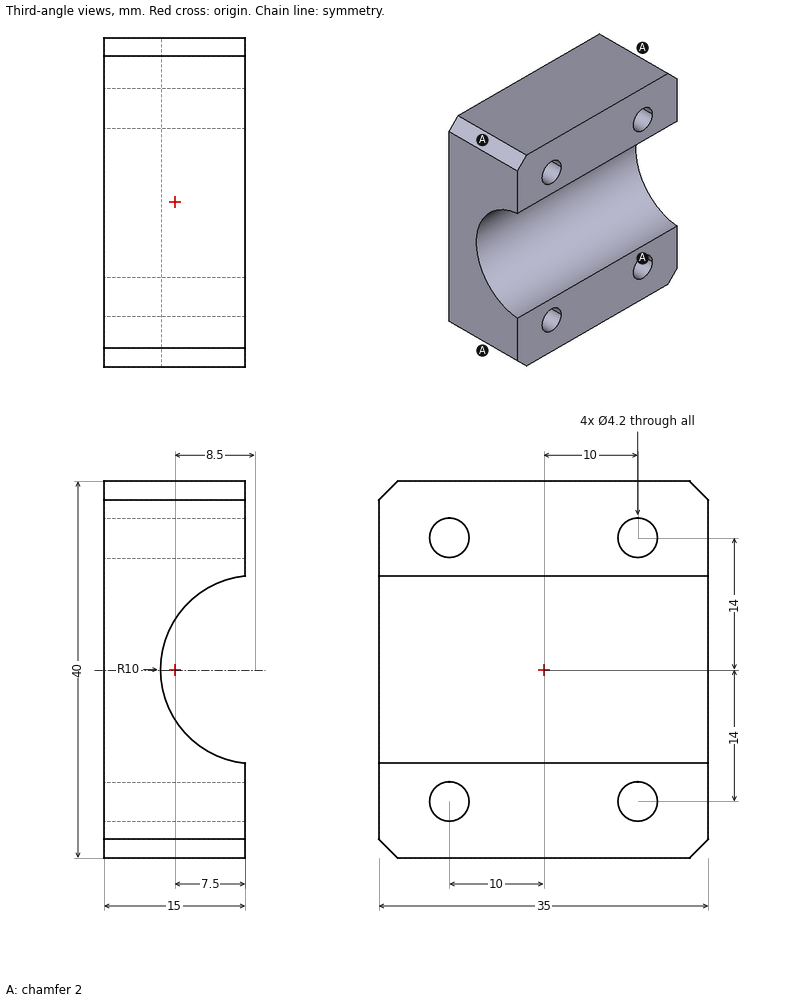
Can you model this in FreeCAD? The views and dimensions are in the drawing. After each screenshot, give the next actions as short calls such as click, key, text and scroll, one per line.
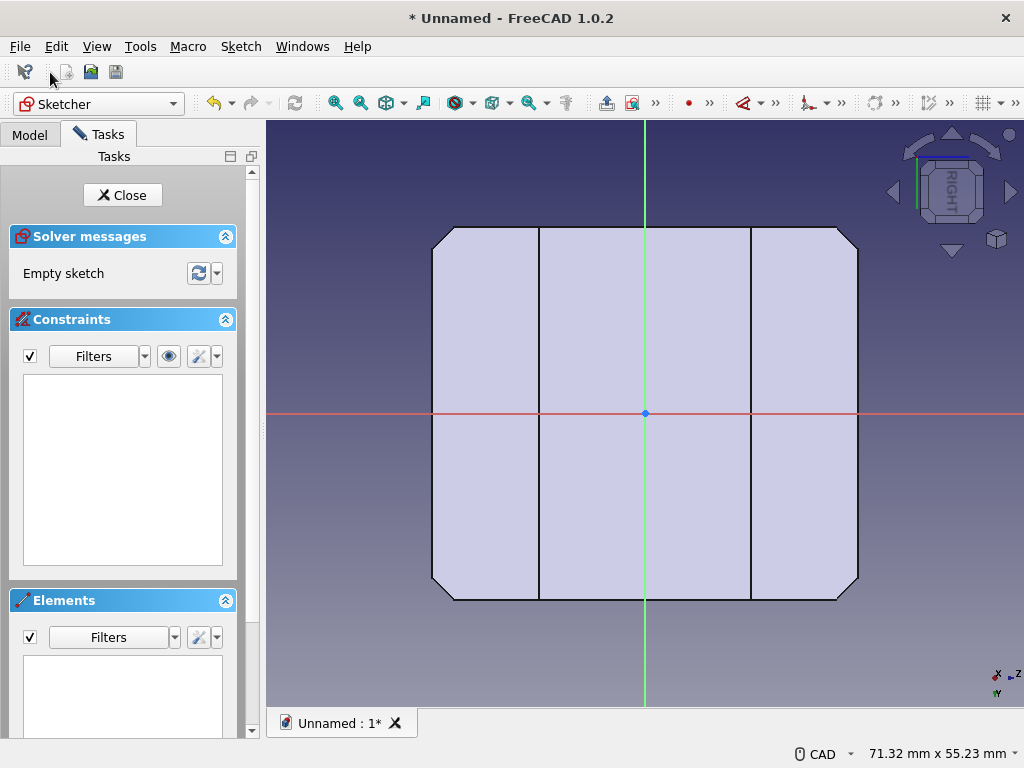
key(g)
key(c)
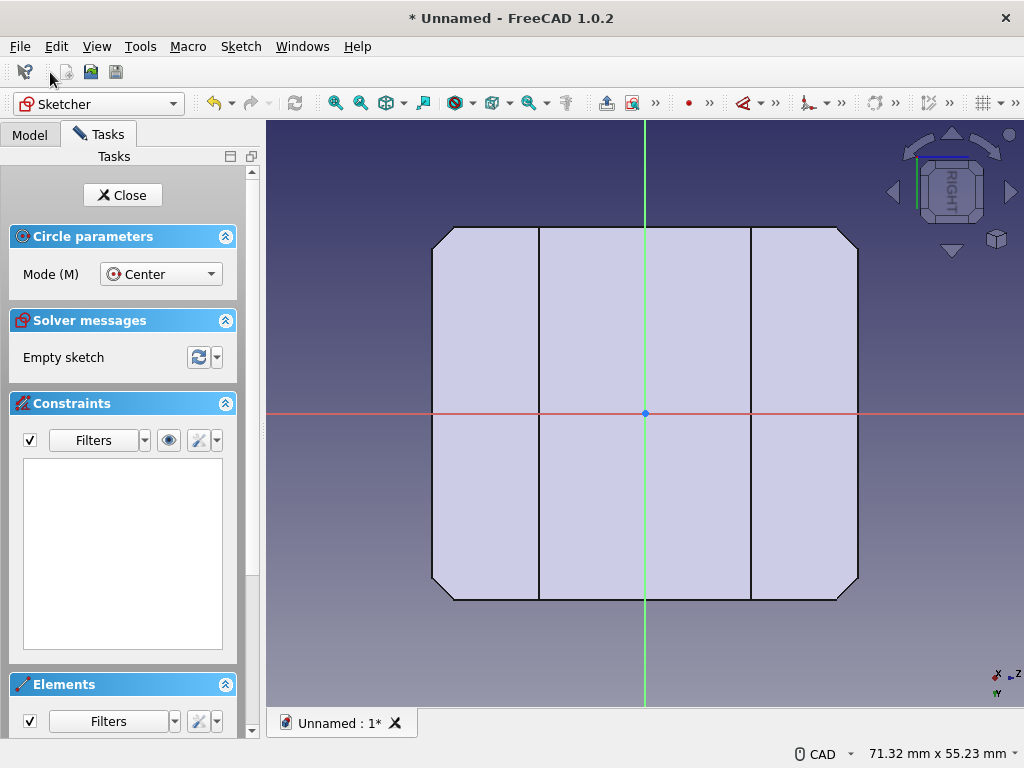
click(794, 520)
move(810, 504)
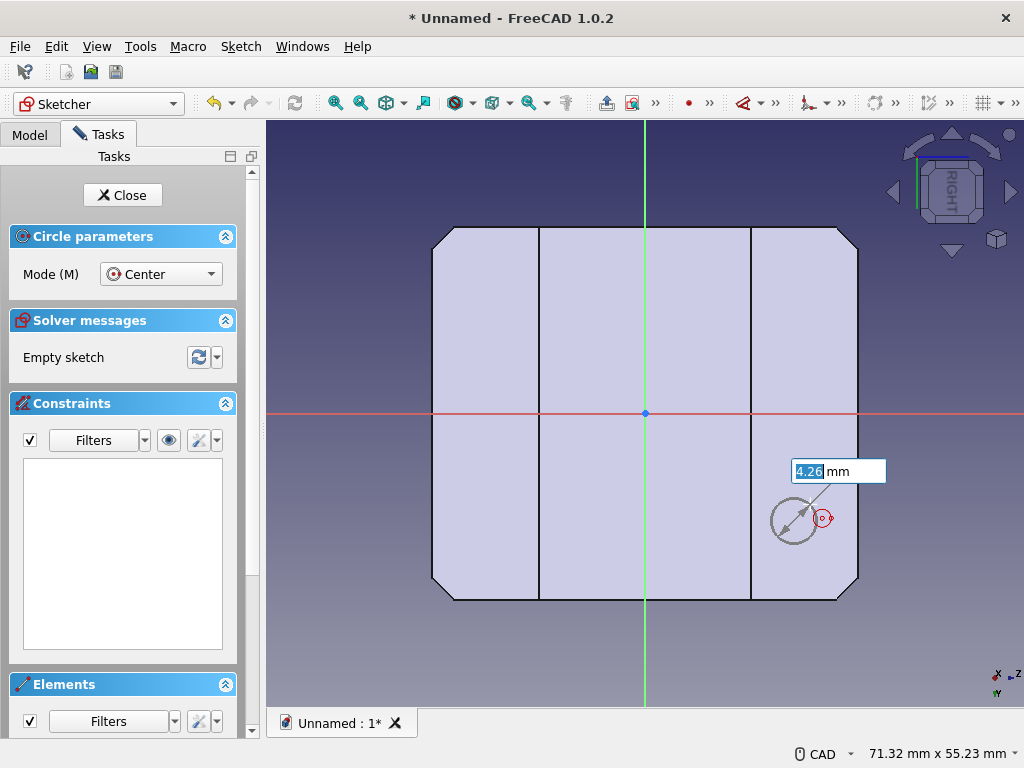
text(4.2)
key(Return)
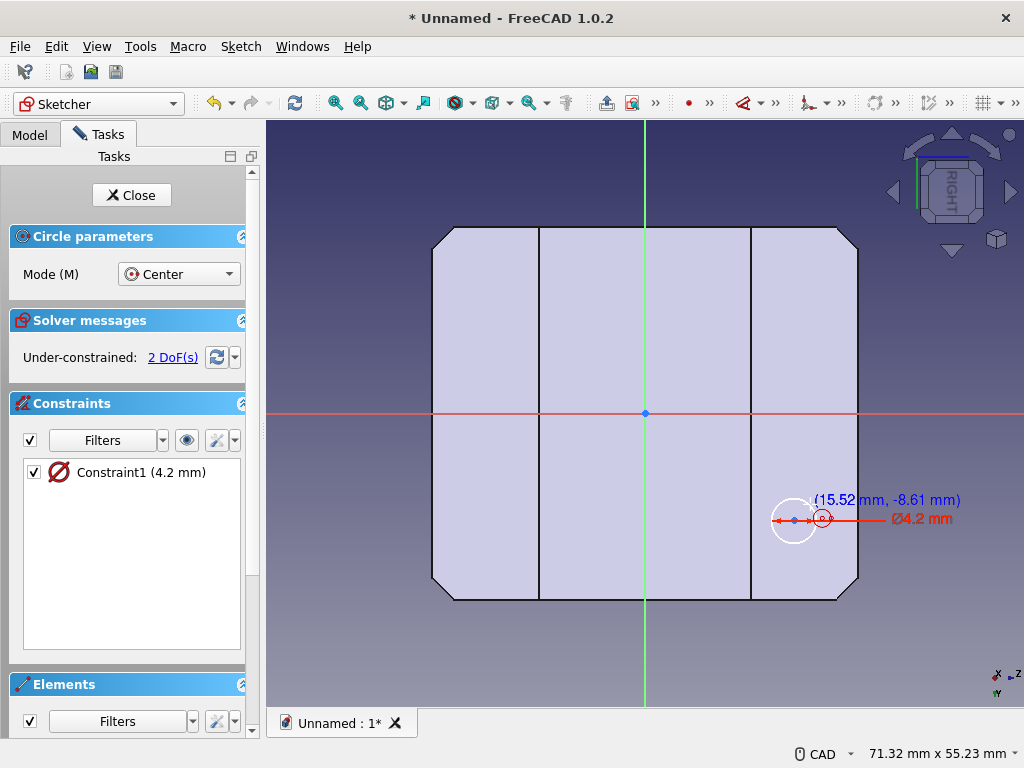
click(496, 520)
move(512, 504)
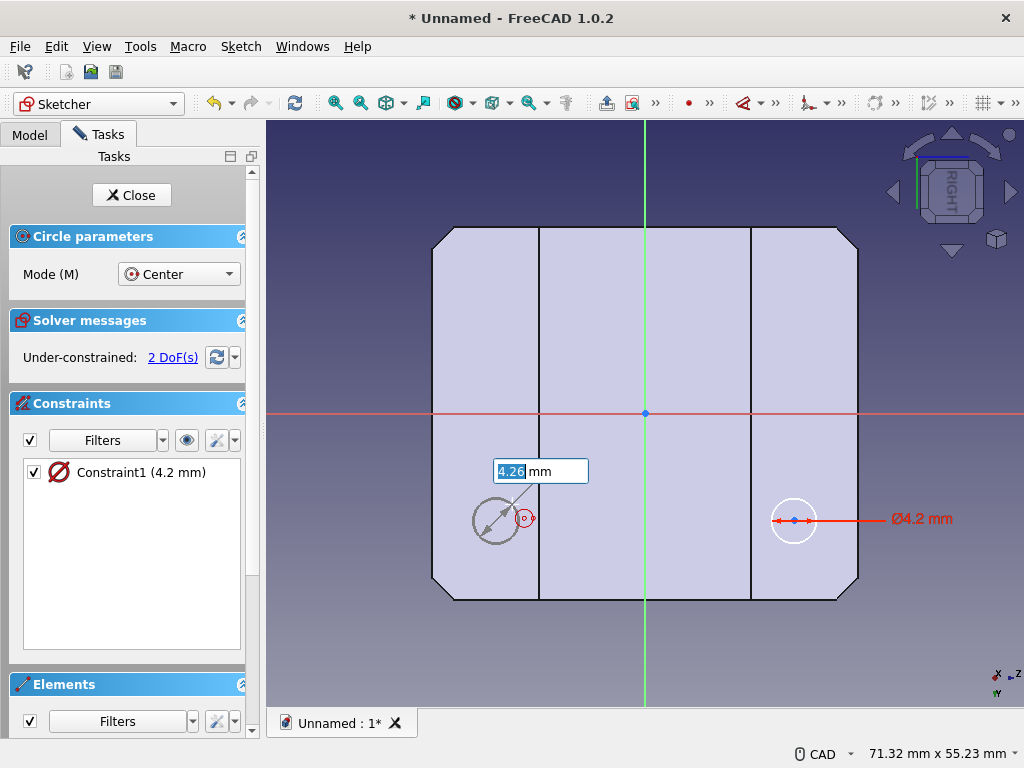
text(4.2)
key(Return)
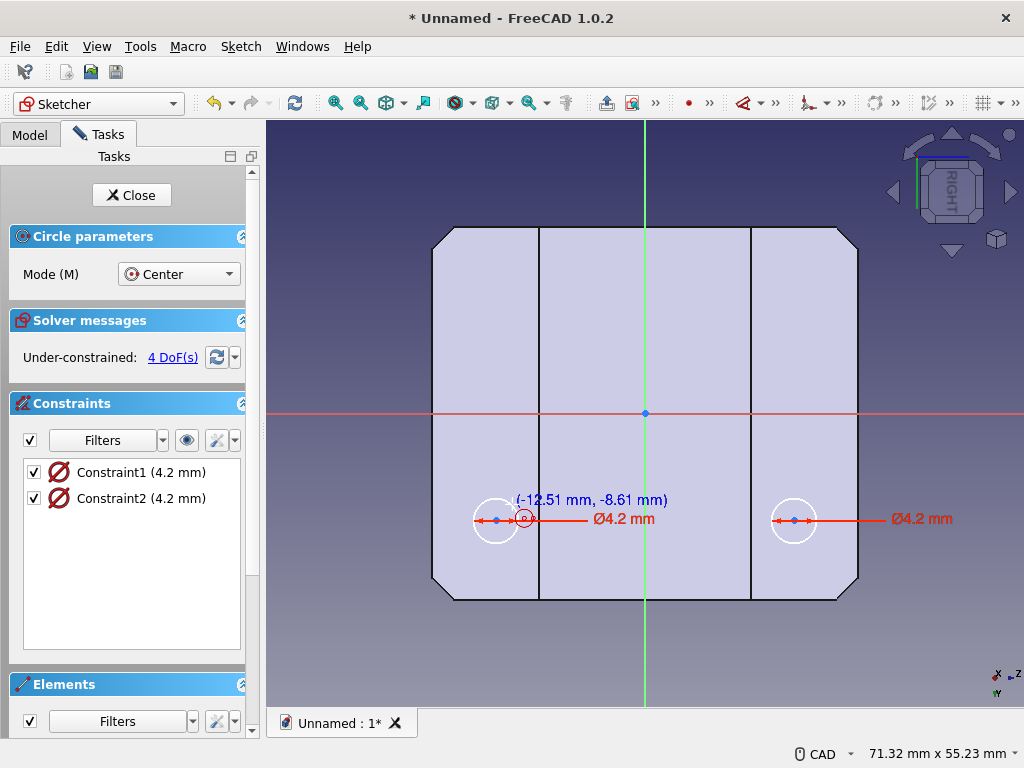
click(496, 307)
move(512, 291)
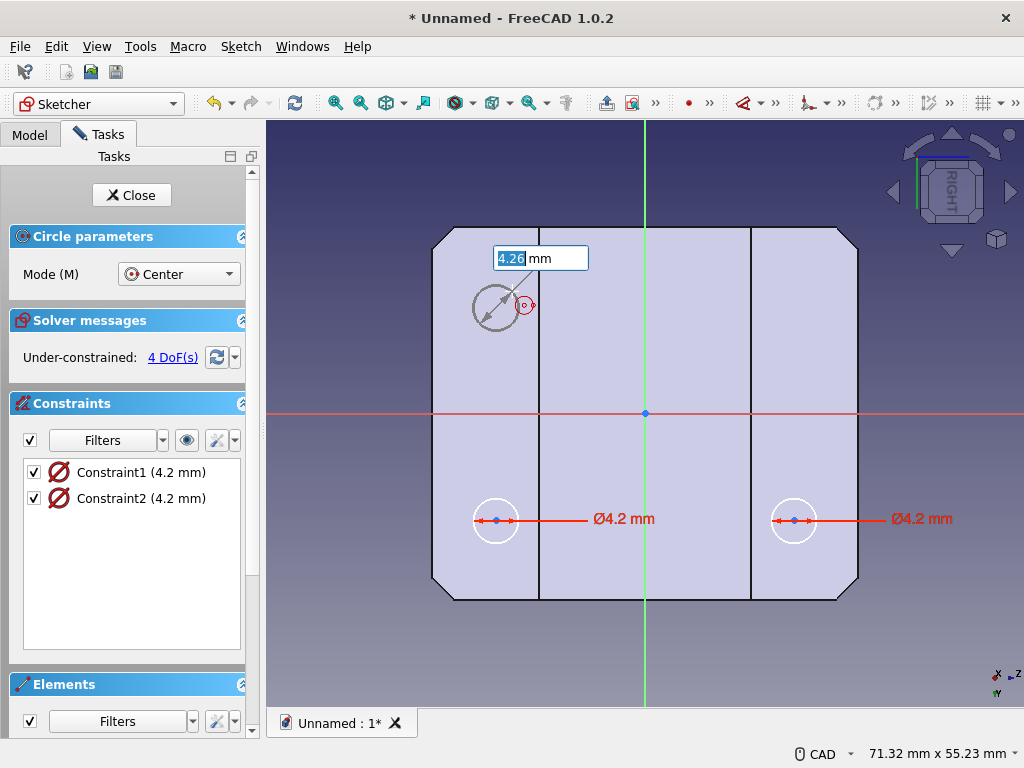
text(4.2)
key(Return)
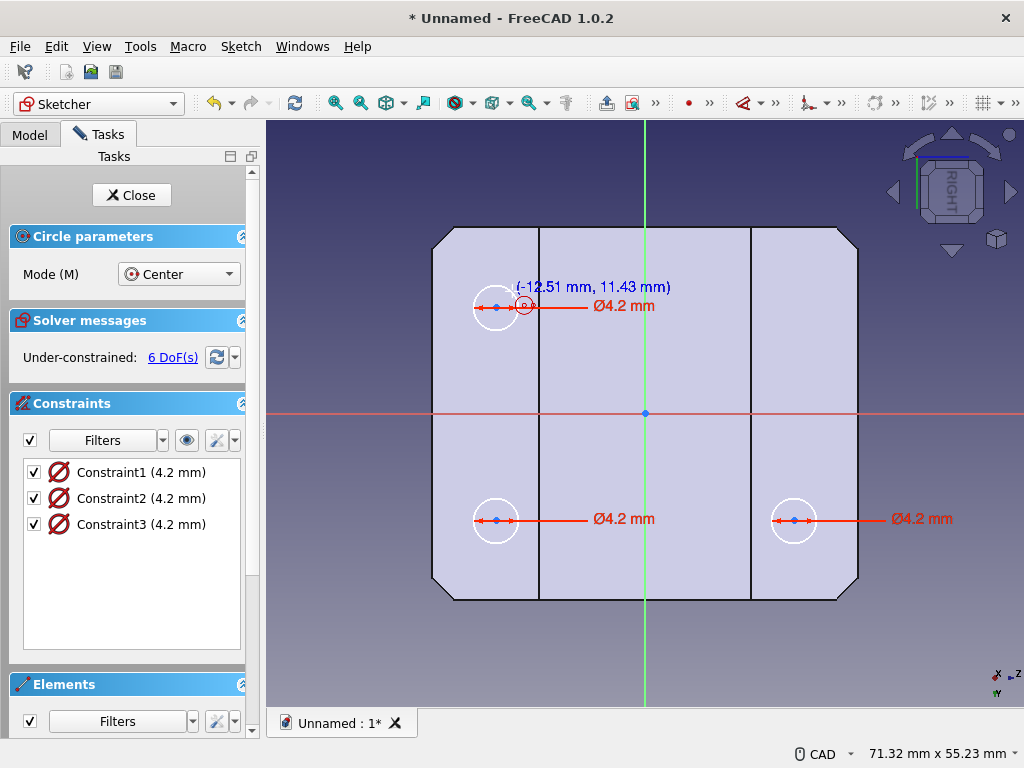
click(794, 307)
move(810, 291)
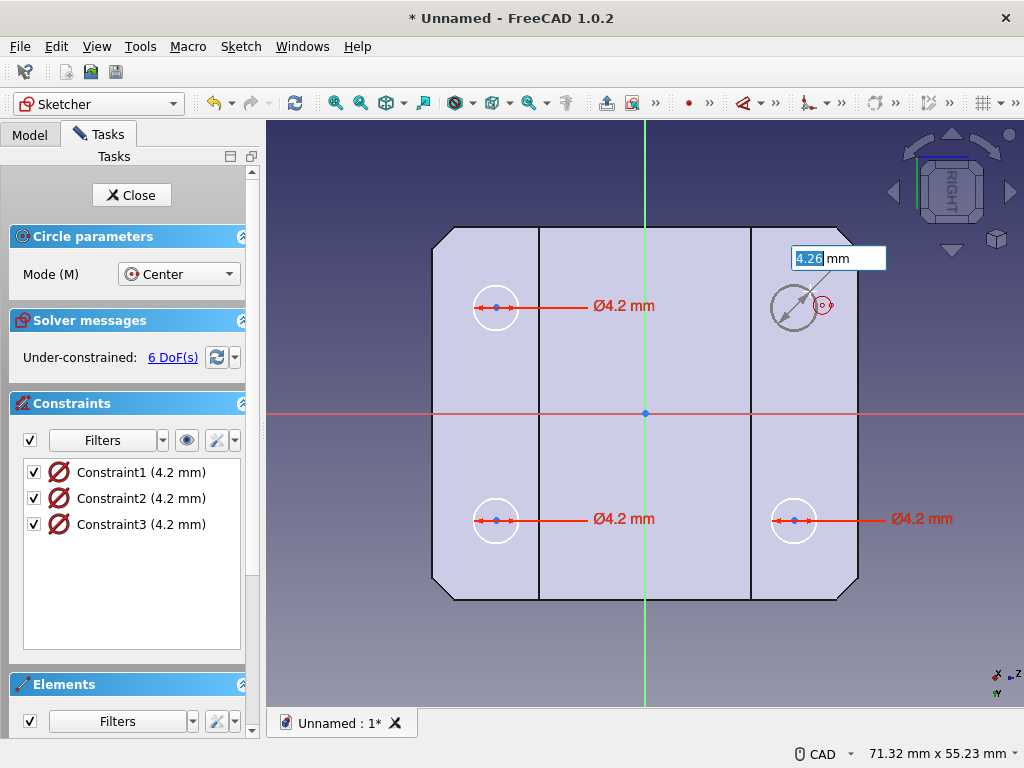
text(4.2)
key(Return)
key(Escape)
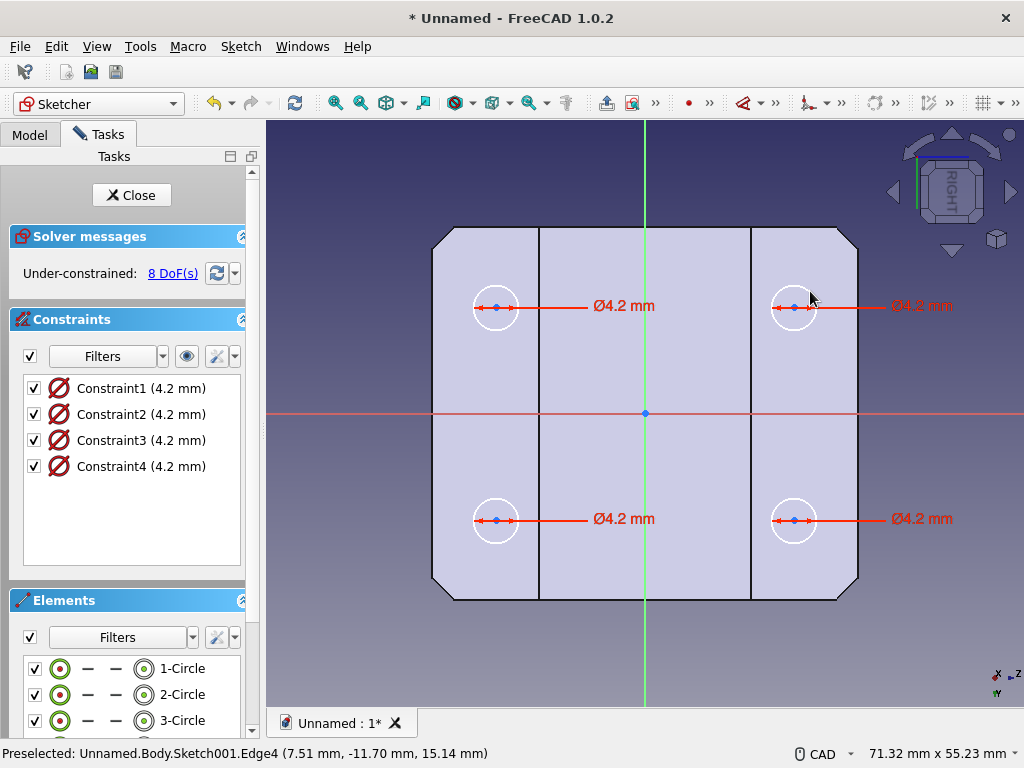
click(794, 521)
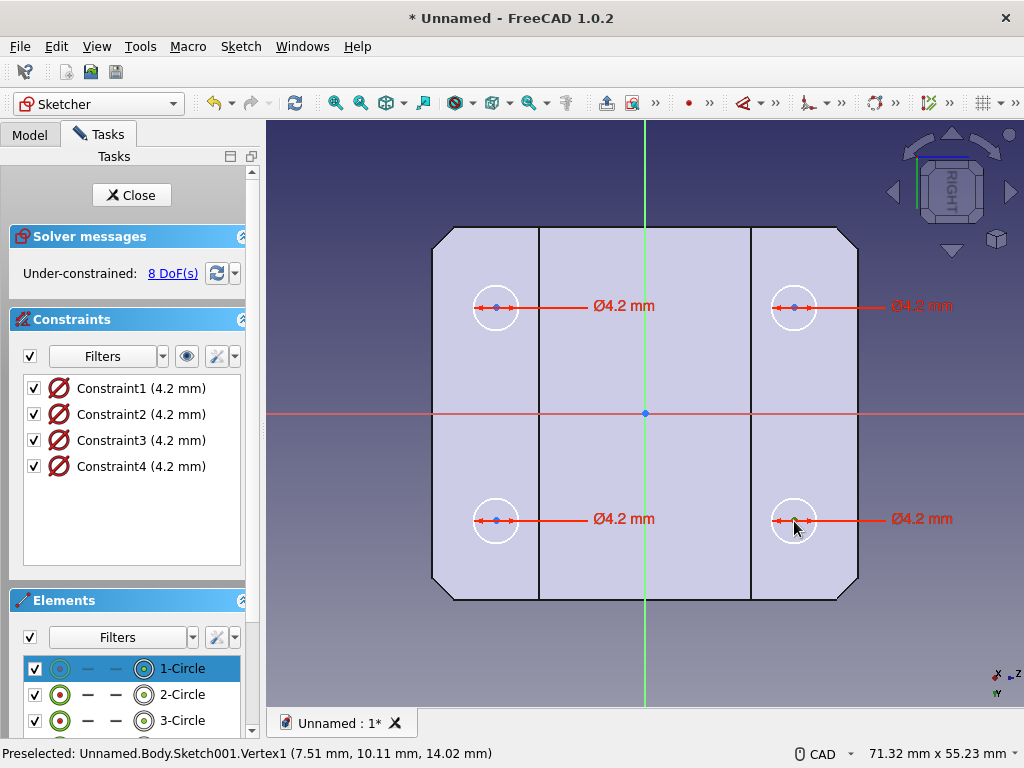
click(496, 521)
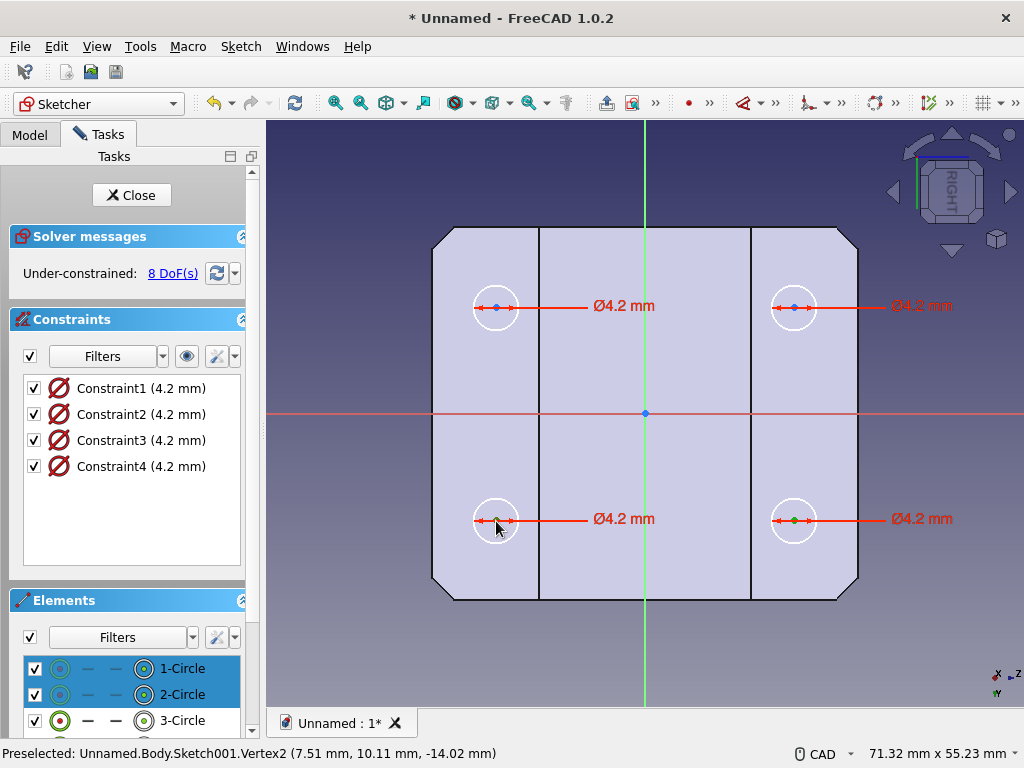
key(h)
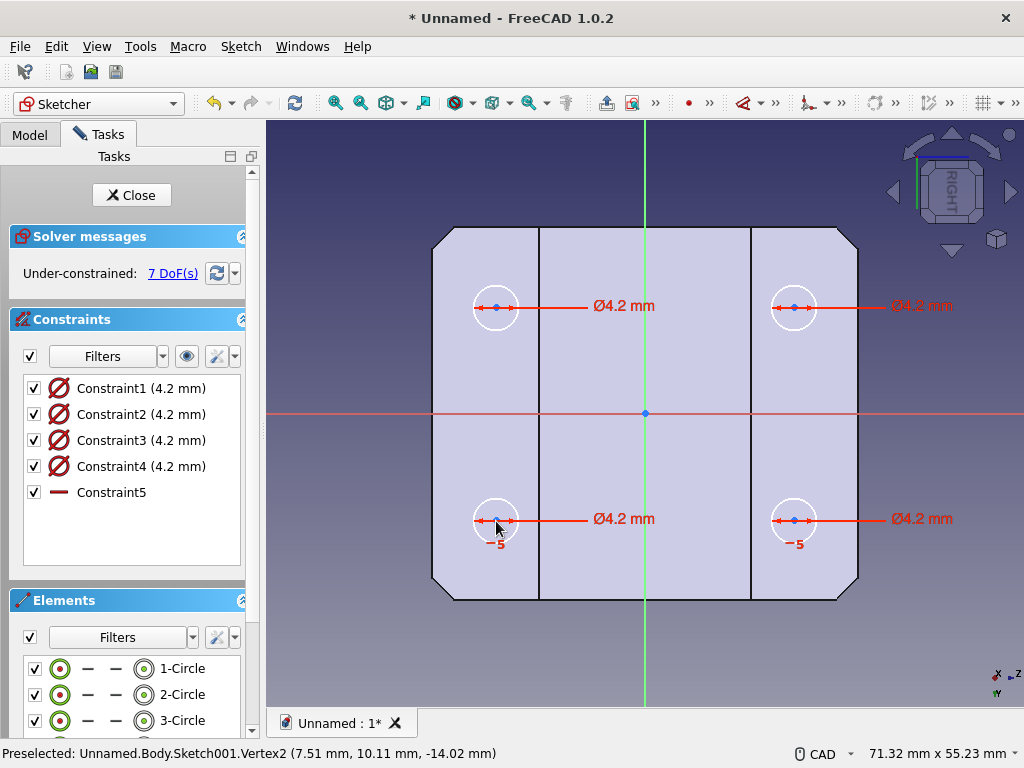
click(496, 521)